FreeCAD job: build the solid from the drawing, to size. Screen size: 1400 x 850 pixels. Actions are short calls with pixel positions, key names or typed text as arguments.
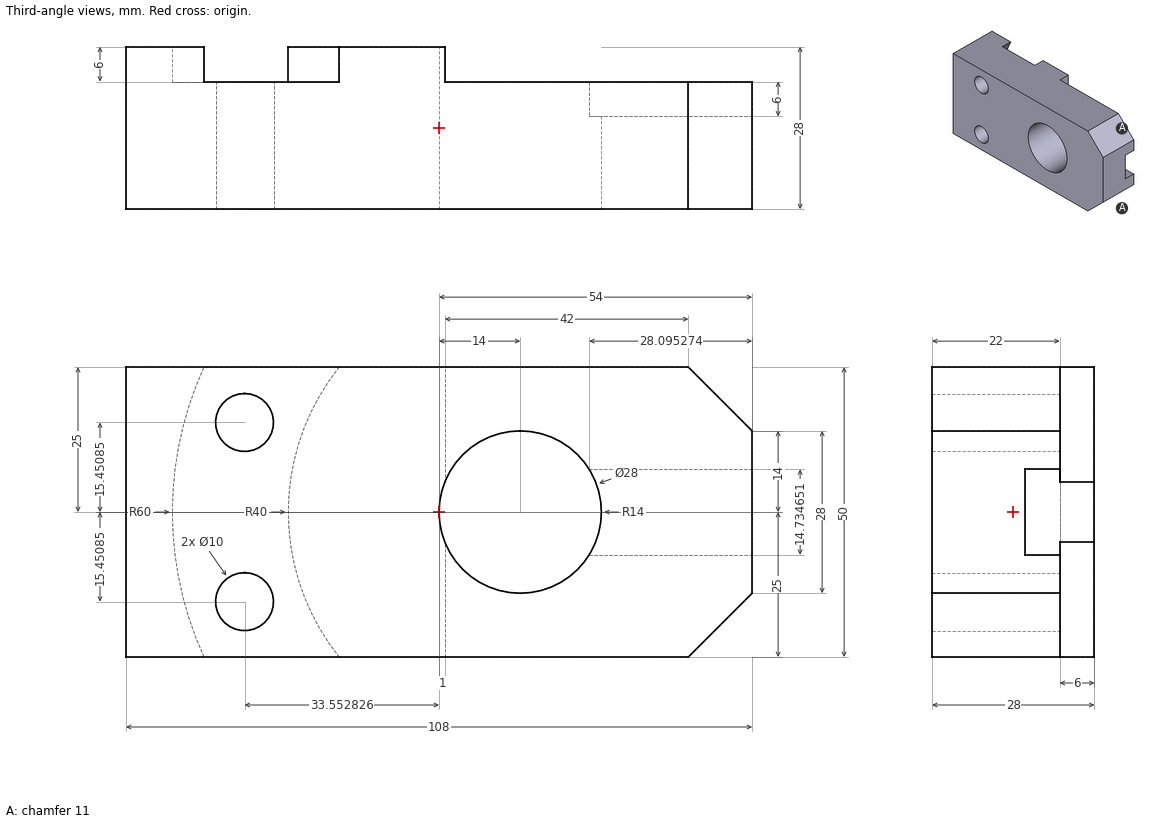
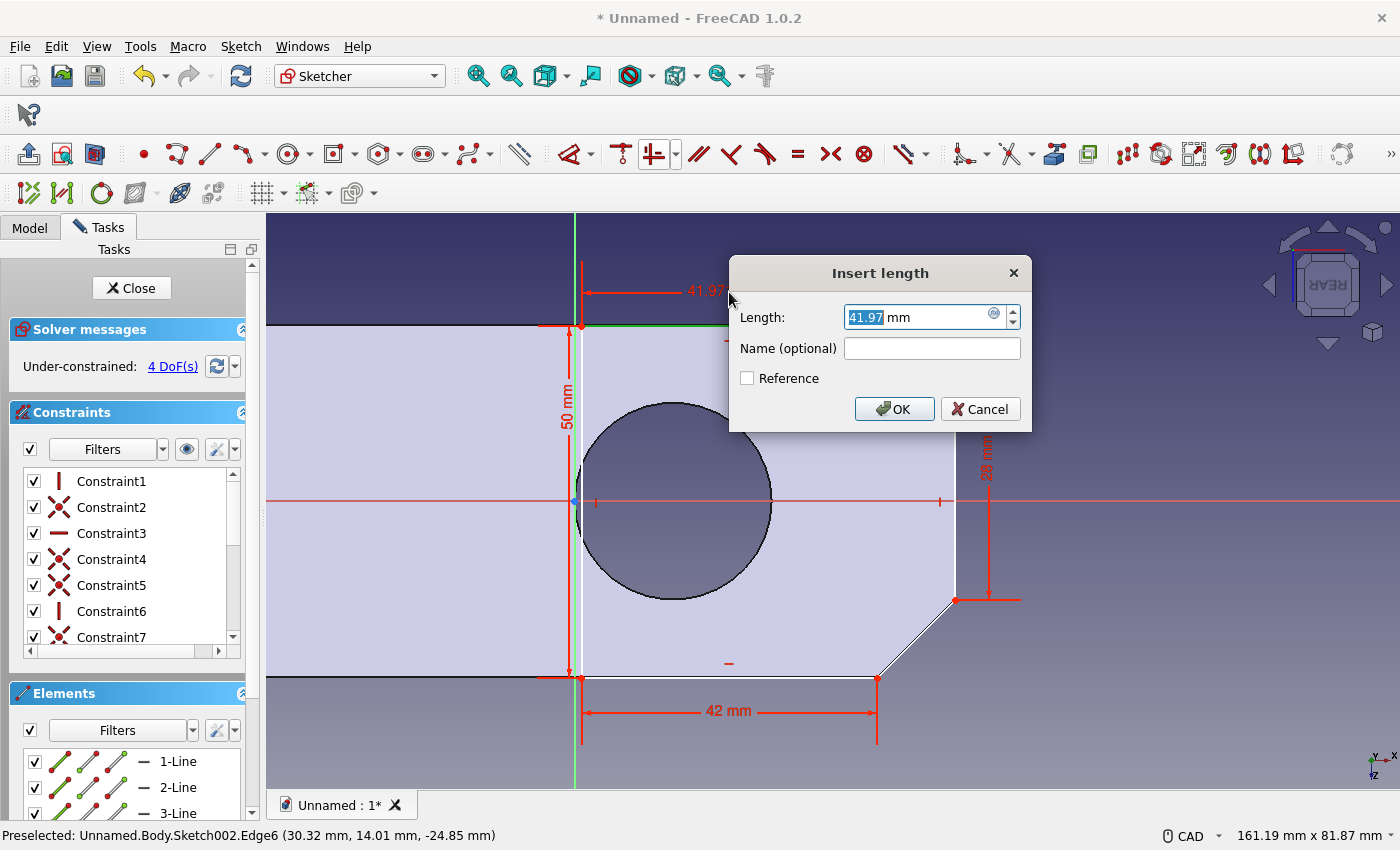
text(42)
key(Return)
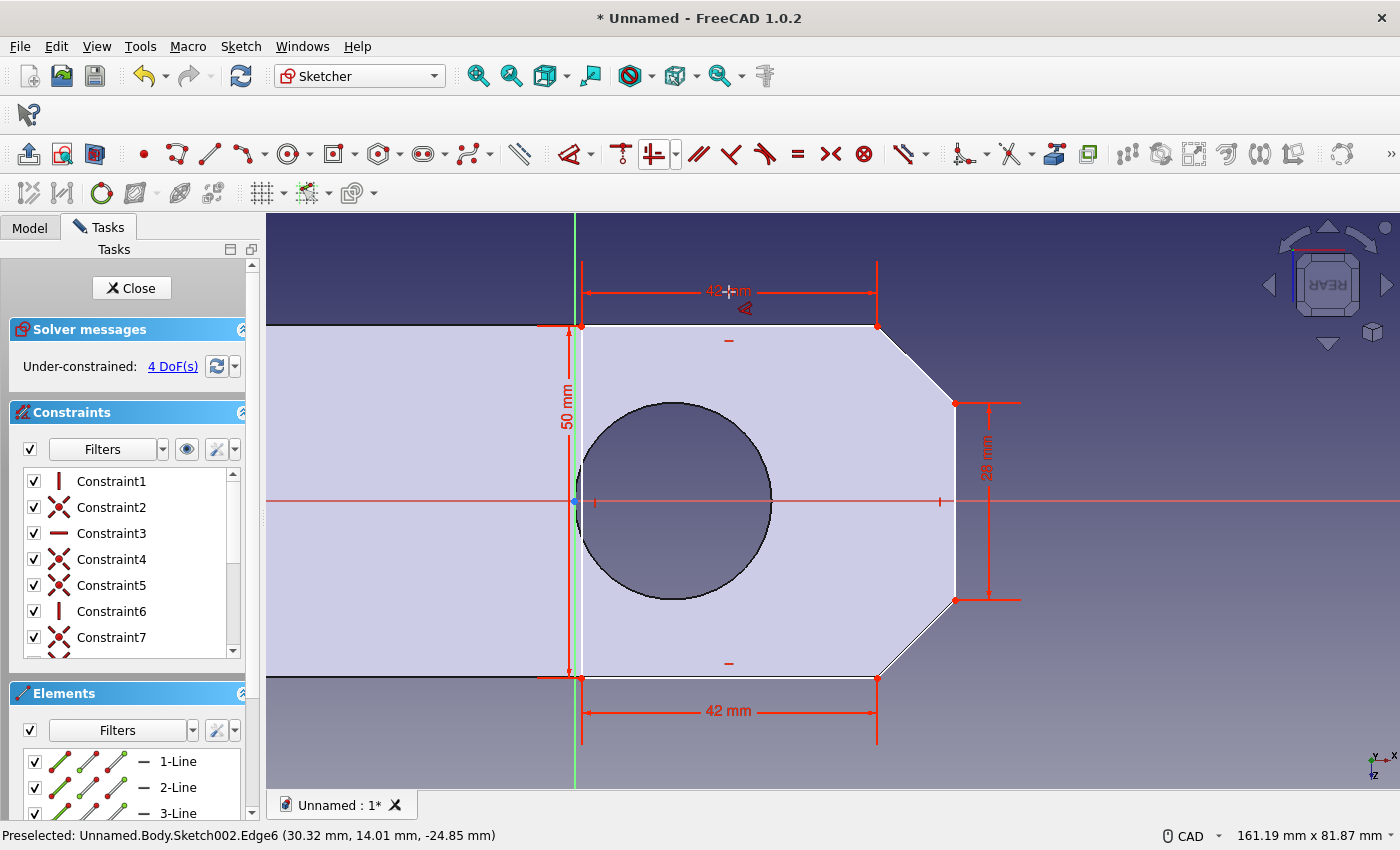
scroll(582, 326, up, 9)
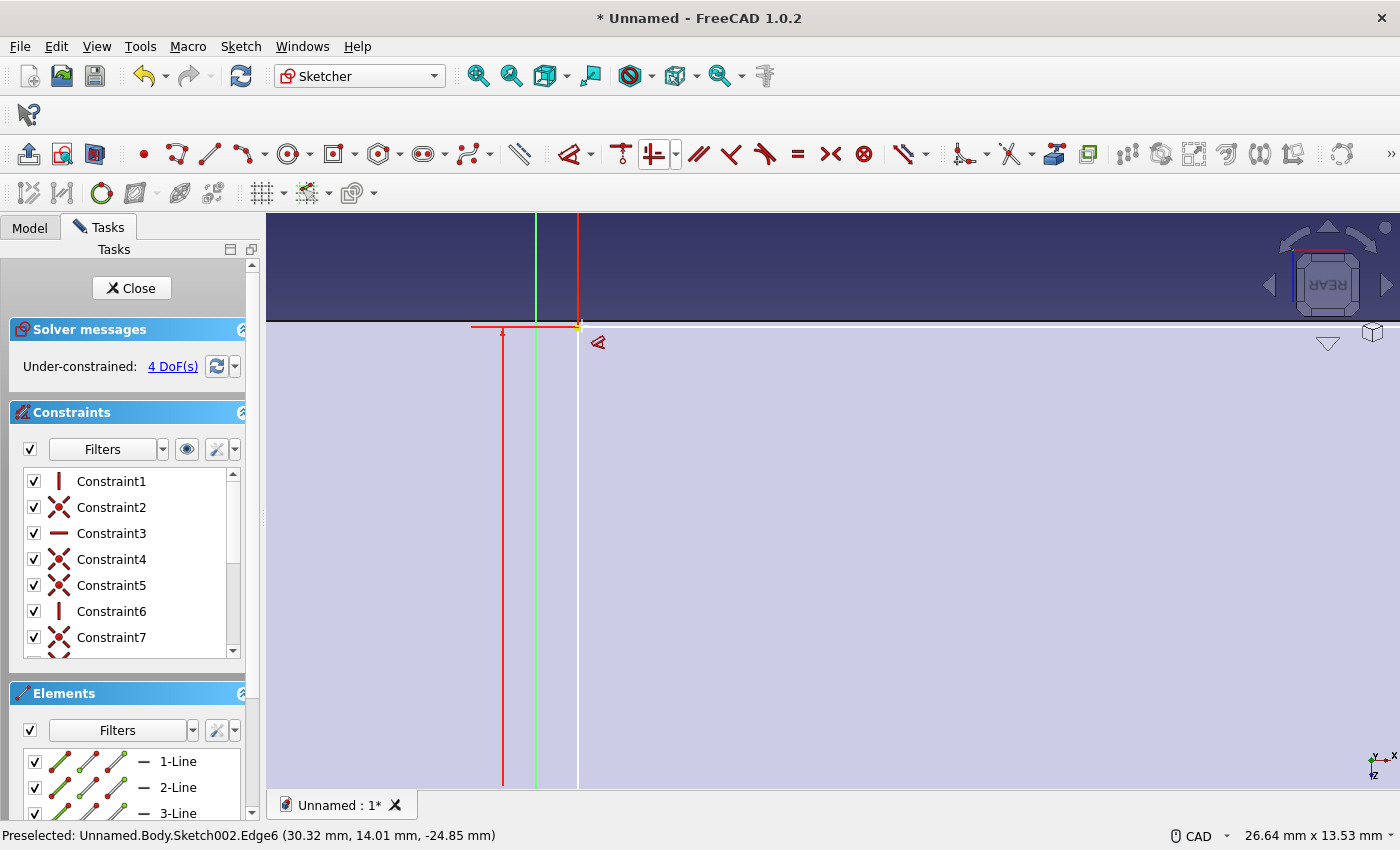
click(578, 327)
click(557, 293)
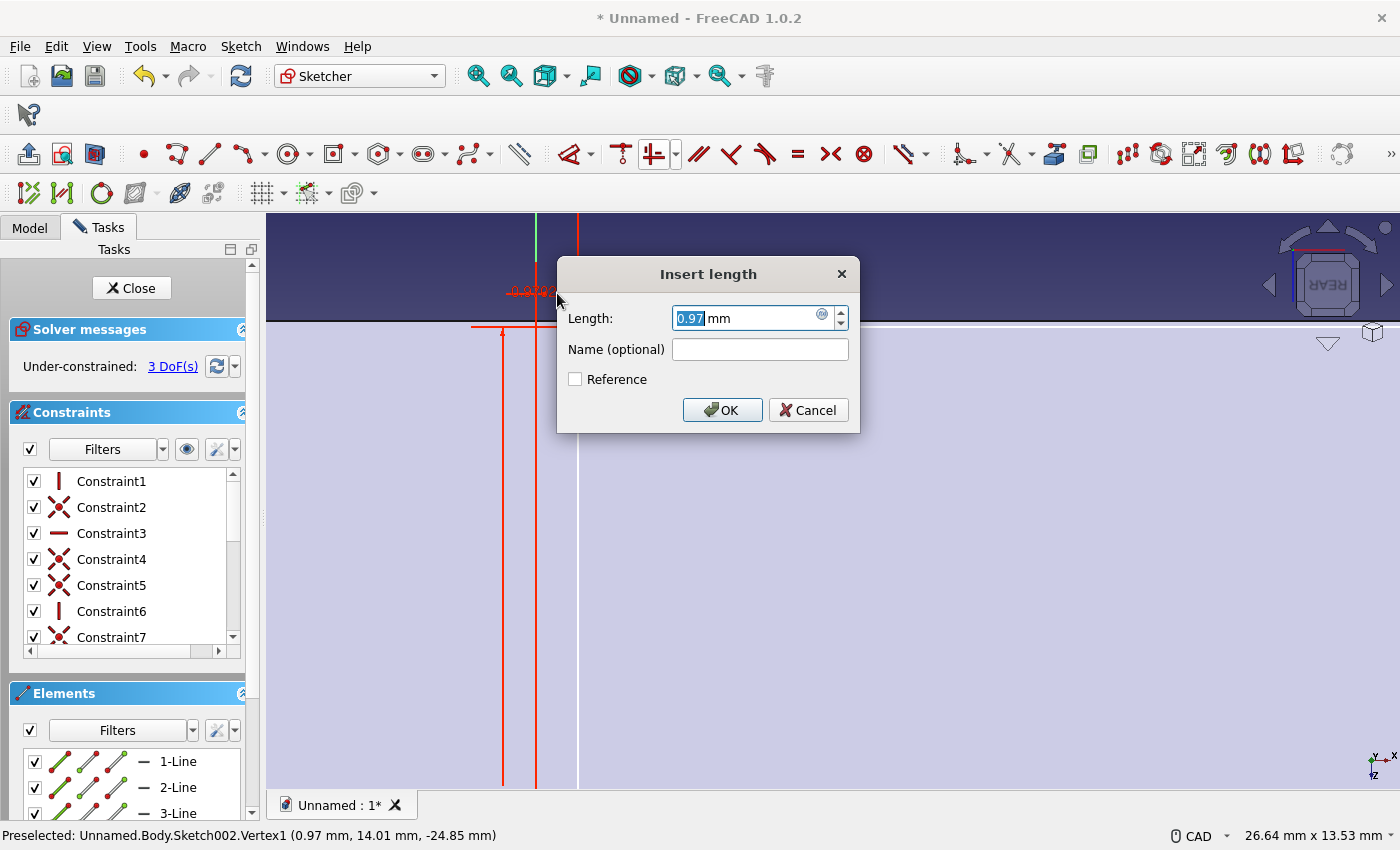
text(1)
key(Return)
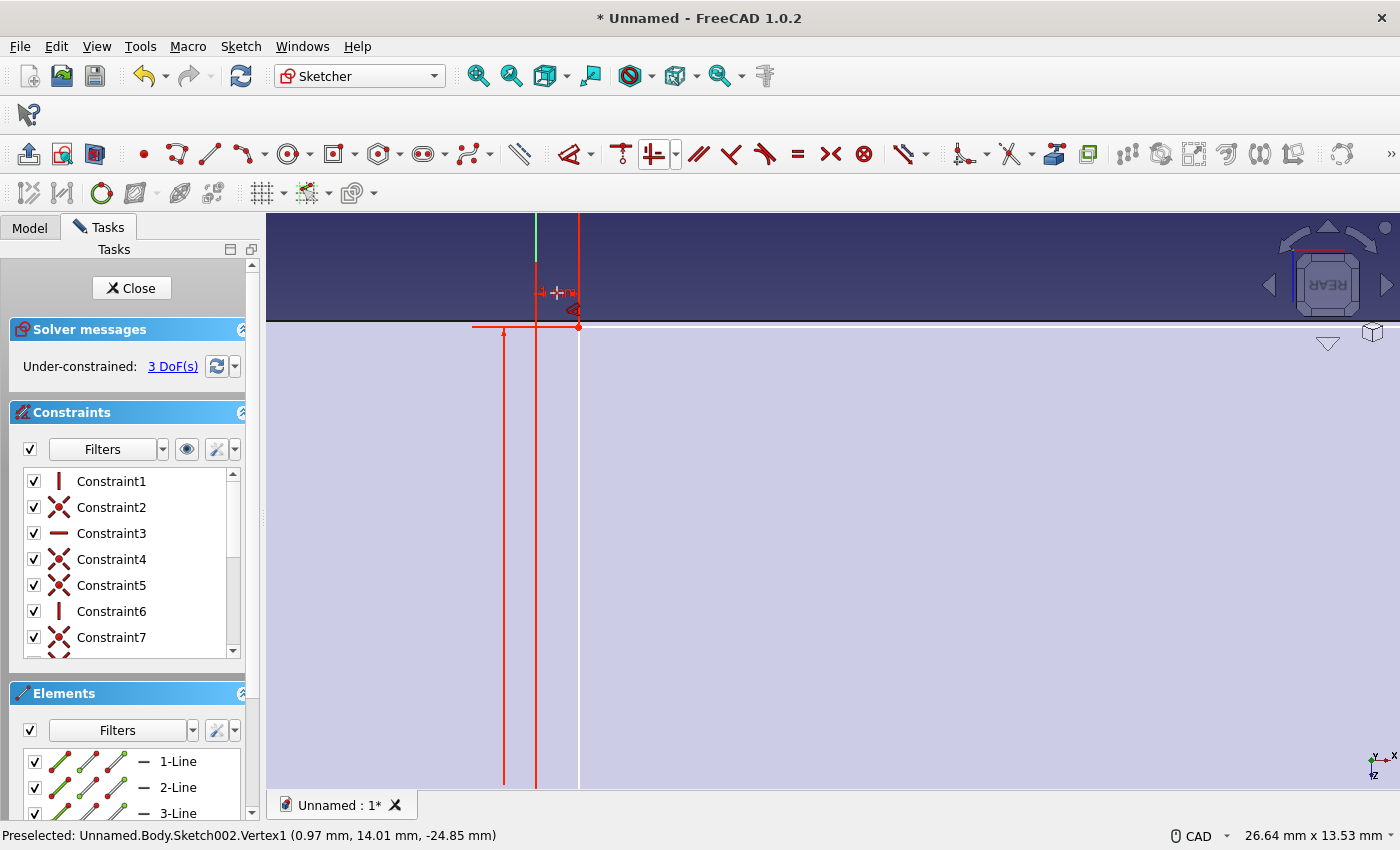
scroll(582, 326, down, 9)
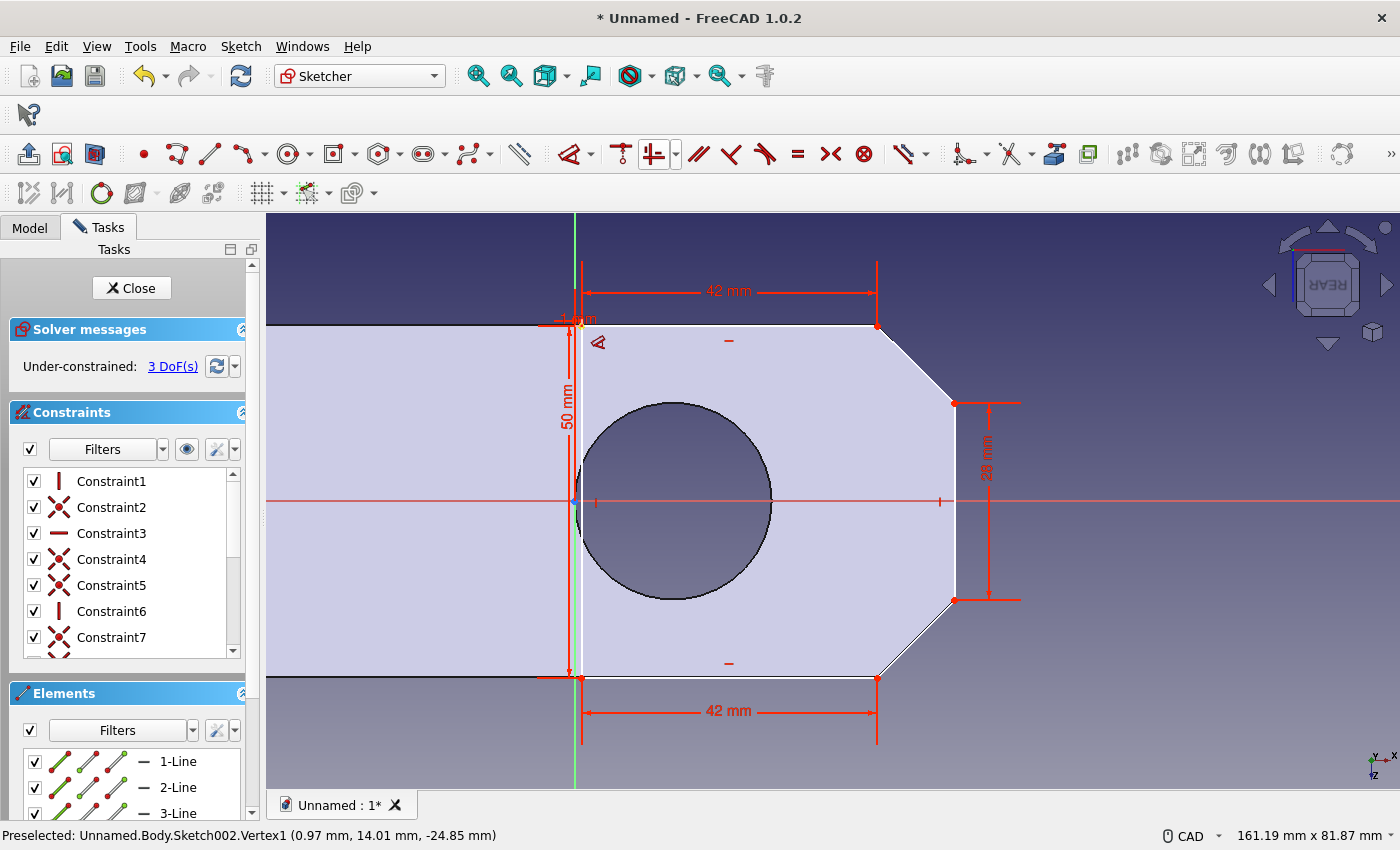
click(582, 326)
click(541, 374)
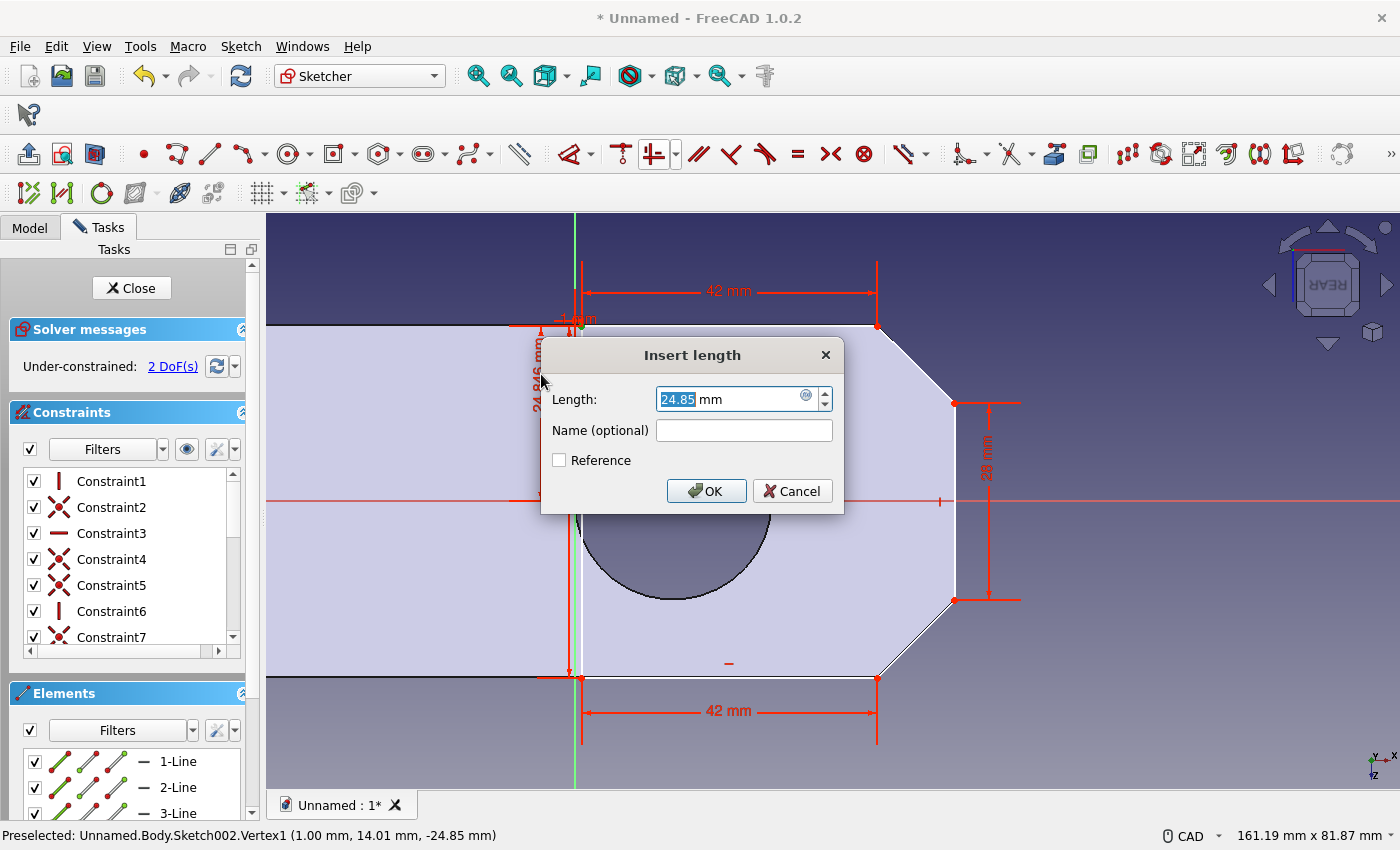
text(25)
key(Return)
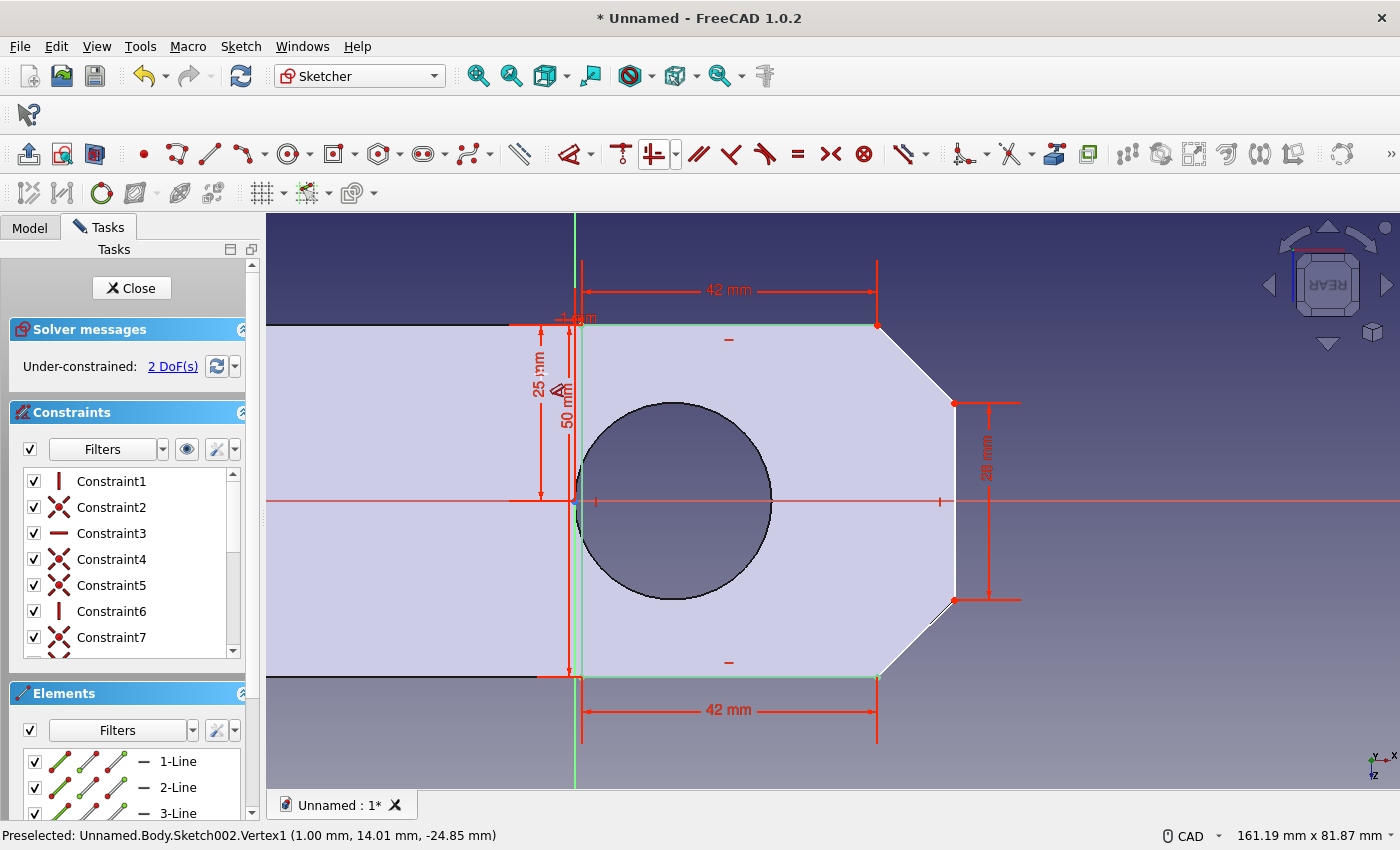
click(955, 600)
click(765, 634)